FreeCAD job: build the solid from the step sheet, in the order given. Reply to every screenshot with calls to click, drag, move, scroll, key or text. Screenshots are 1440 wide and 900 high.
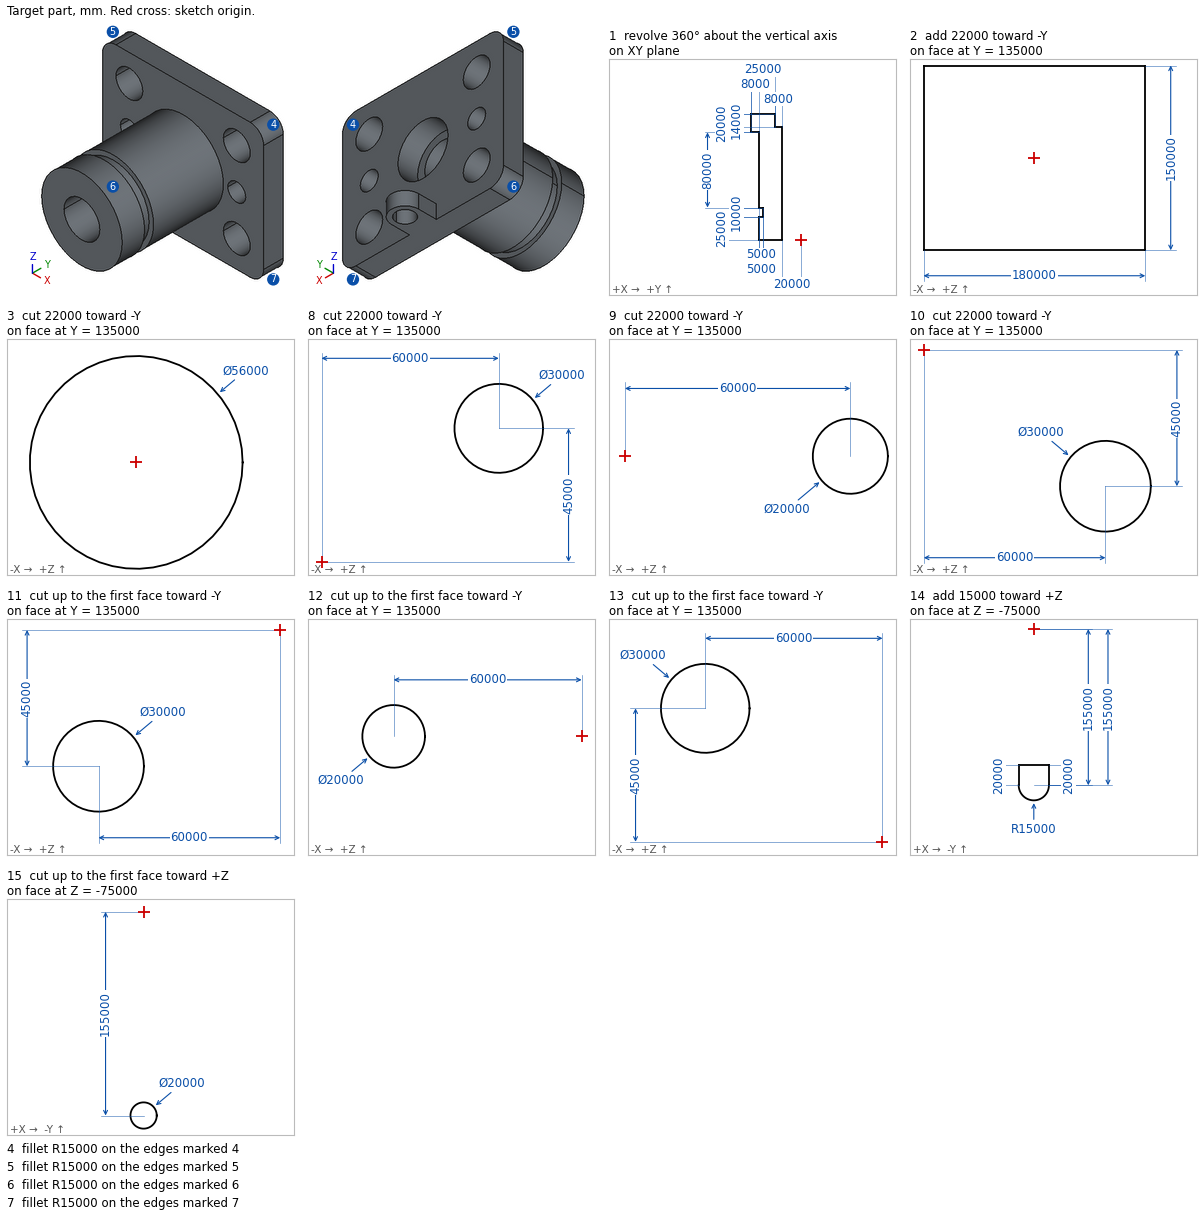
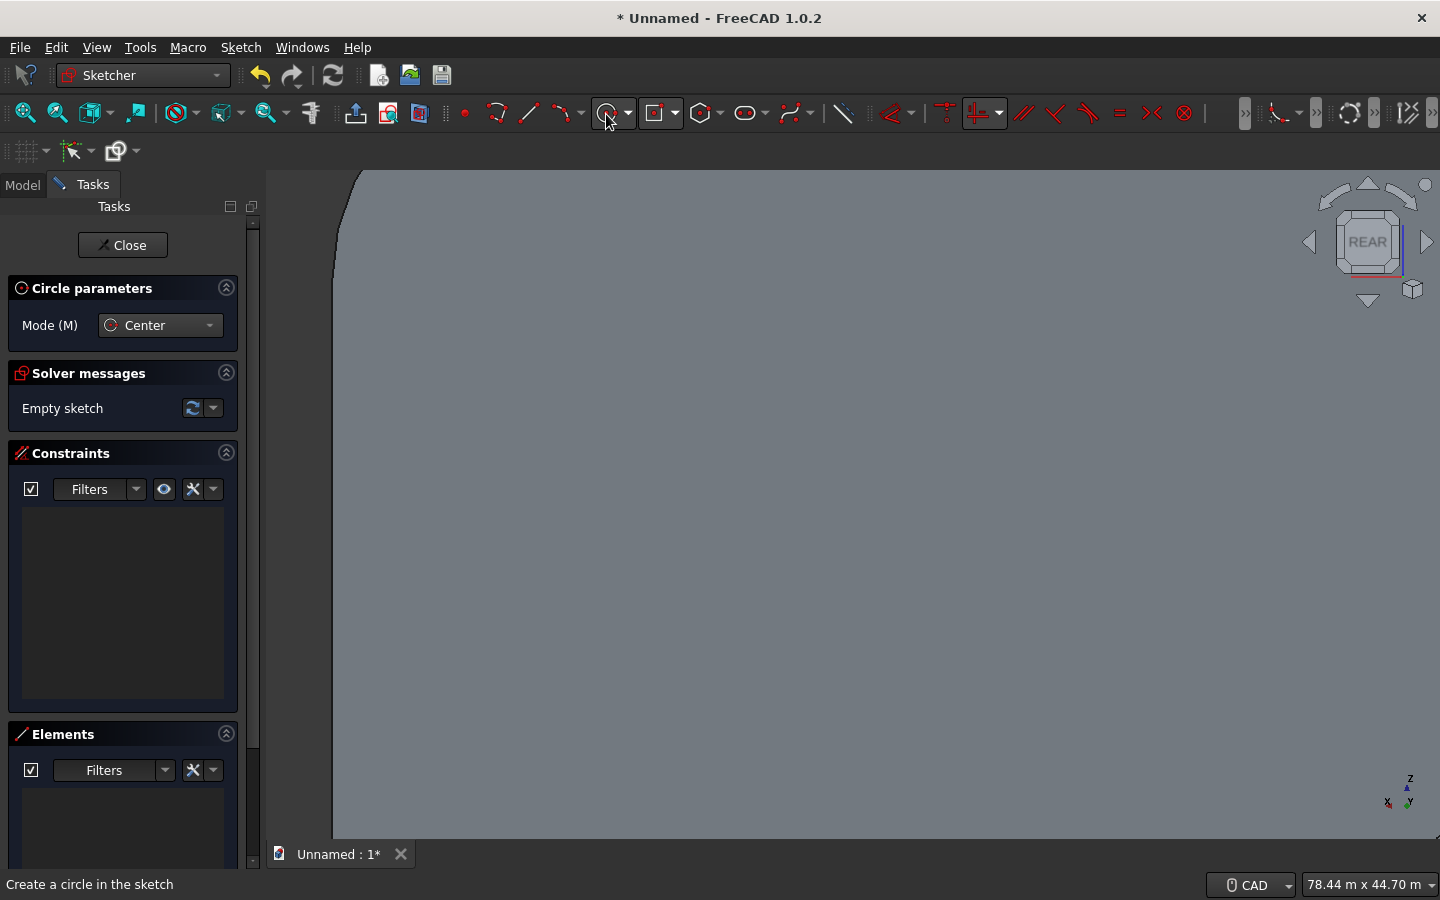
click(781, 504)
click(940, 345)
key(Escape)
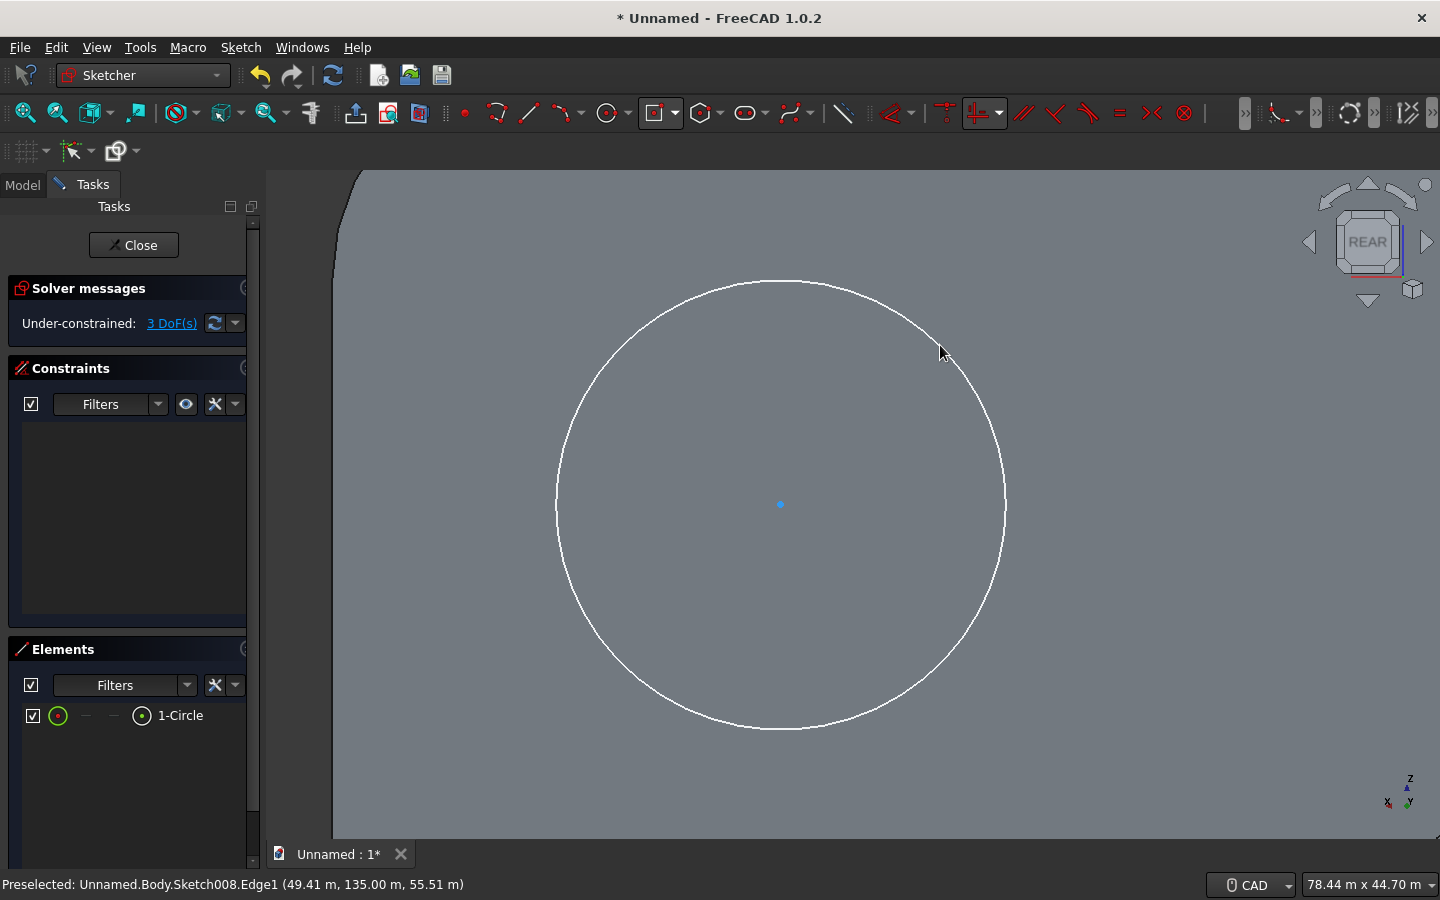
click(890, 114)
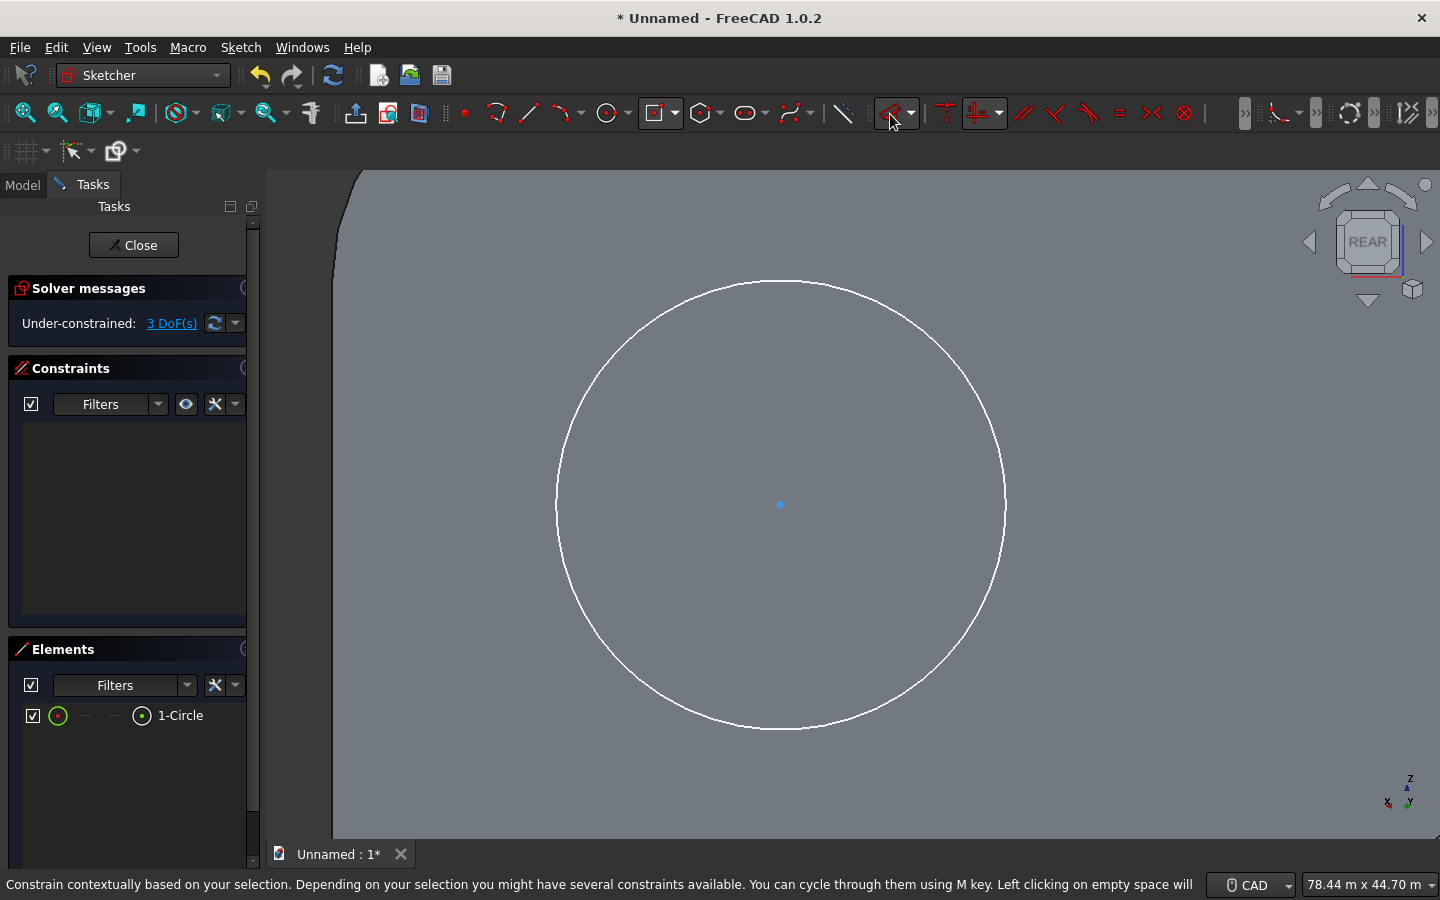
click(940, 346)
click(963, 323)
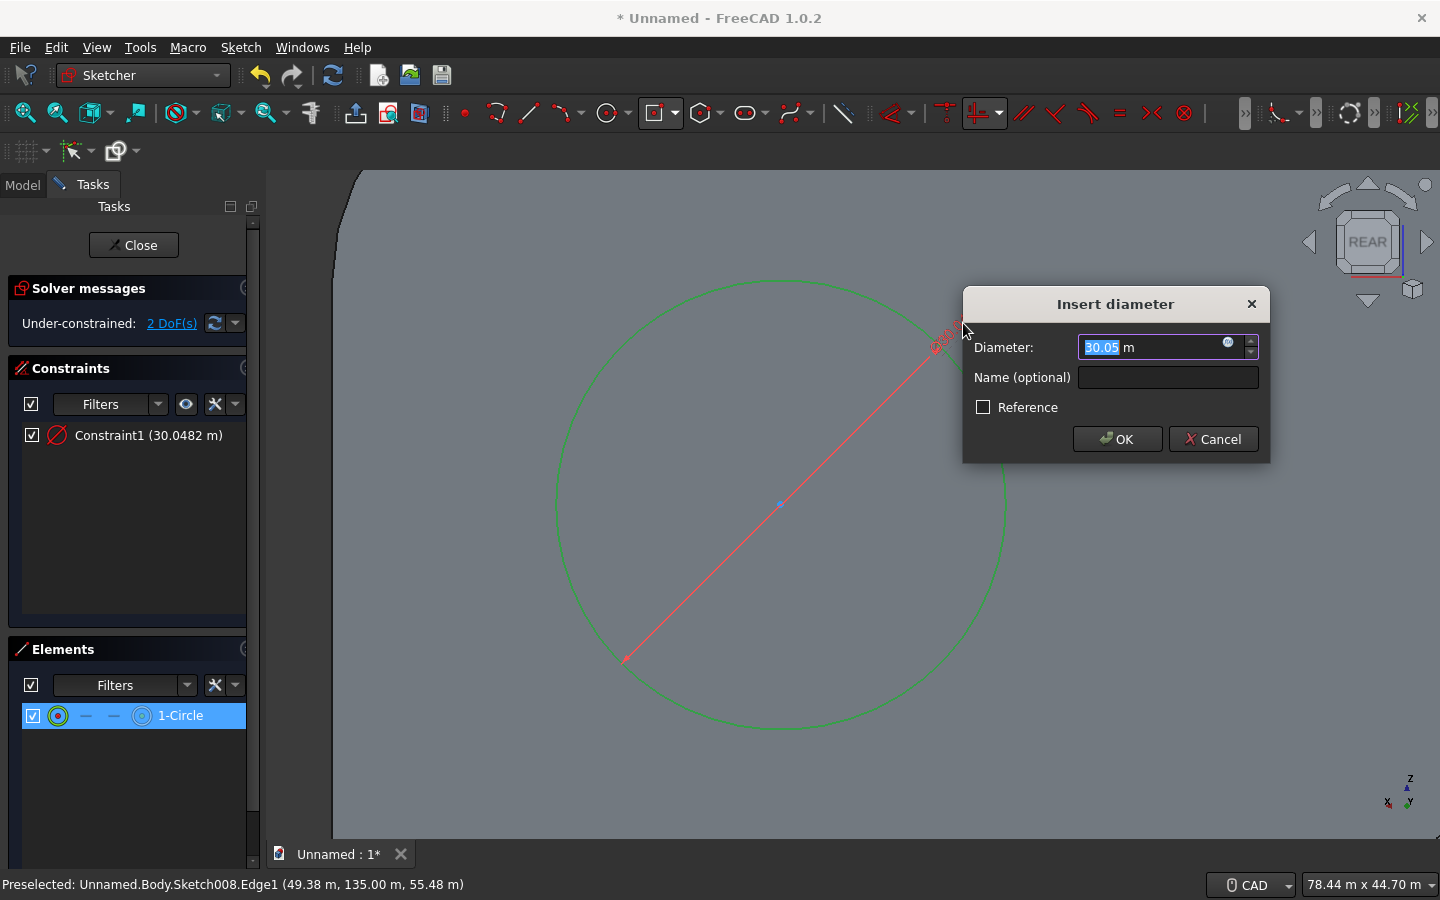
key(ctrl+a)
text(30000 mm)
key(Return)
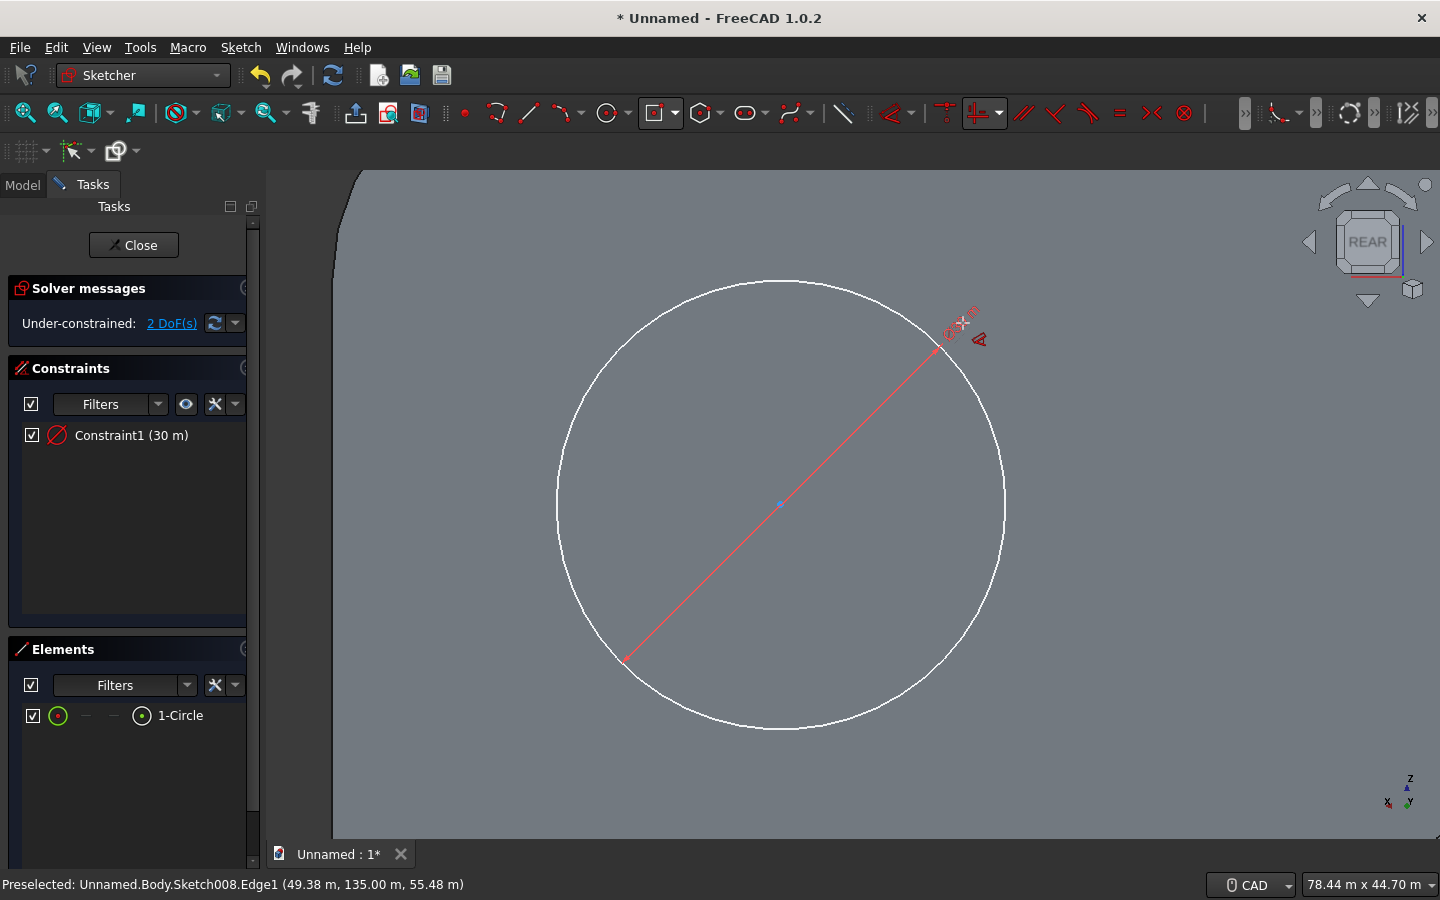
click(781, 505)
click(1028, 471)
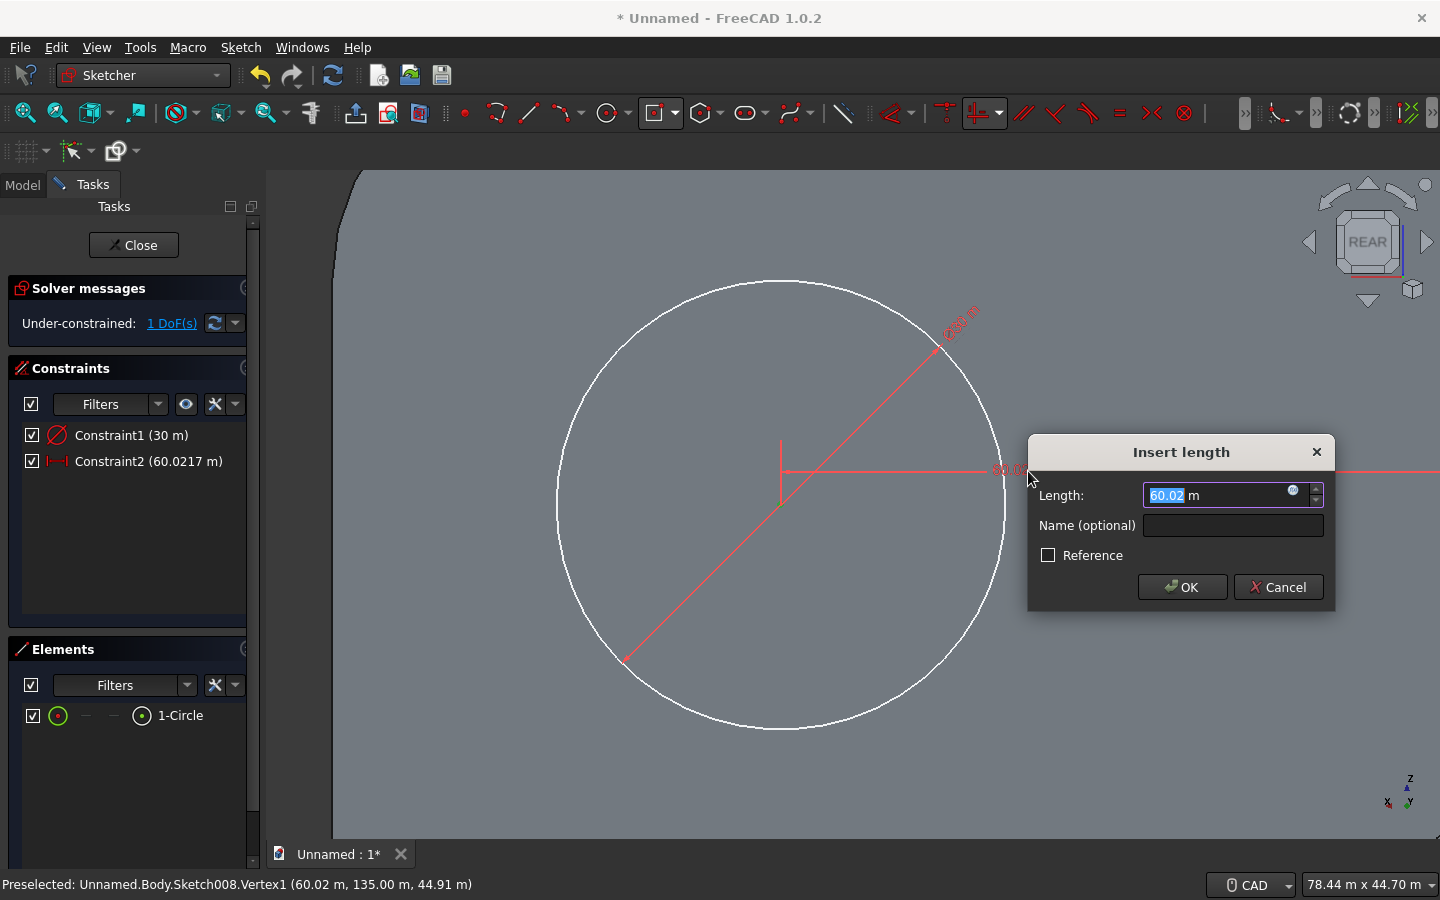
key(ctrl+a)
text(60000 mm)
key(Return)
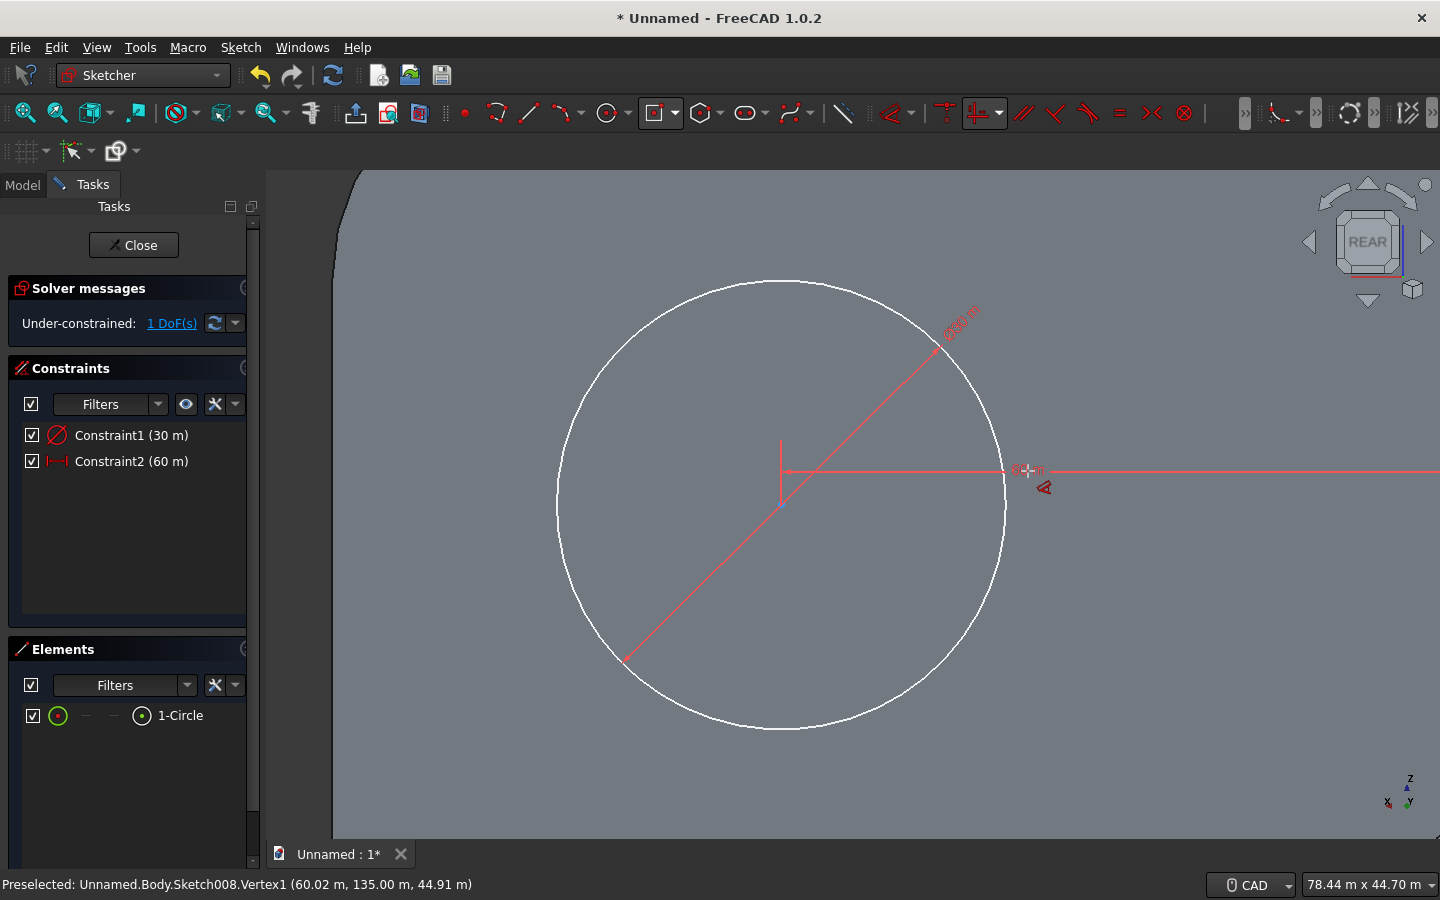
click(781, 505)
click(747, 658)